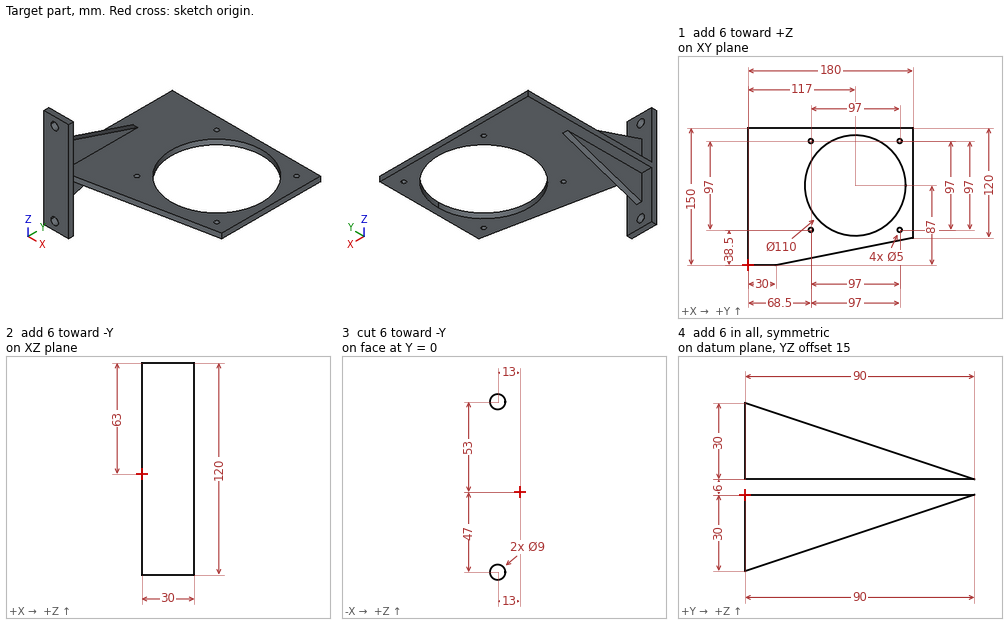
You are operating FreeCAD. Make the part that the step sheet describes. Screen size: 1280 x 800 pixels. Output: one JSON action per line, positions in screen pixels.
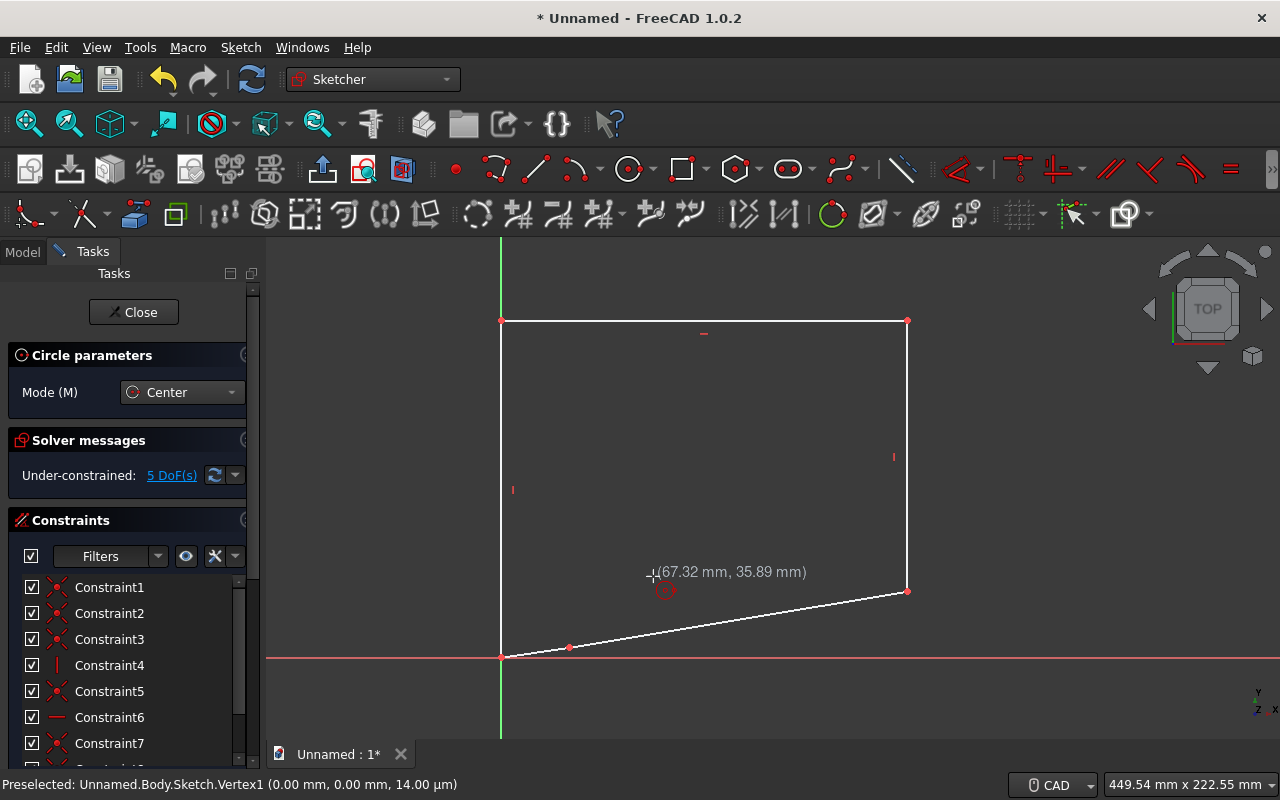
{"action": "left_click", "coordinate": [656, 571]}
{"action": "mouse_move", "coordinate": [660, 567]}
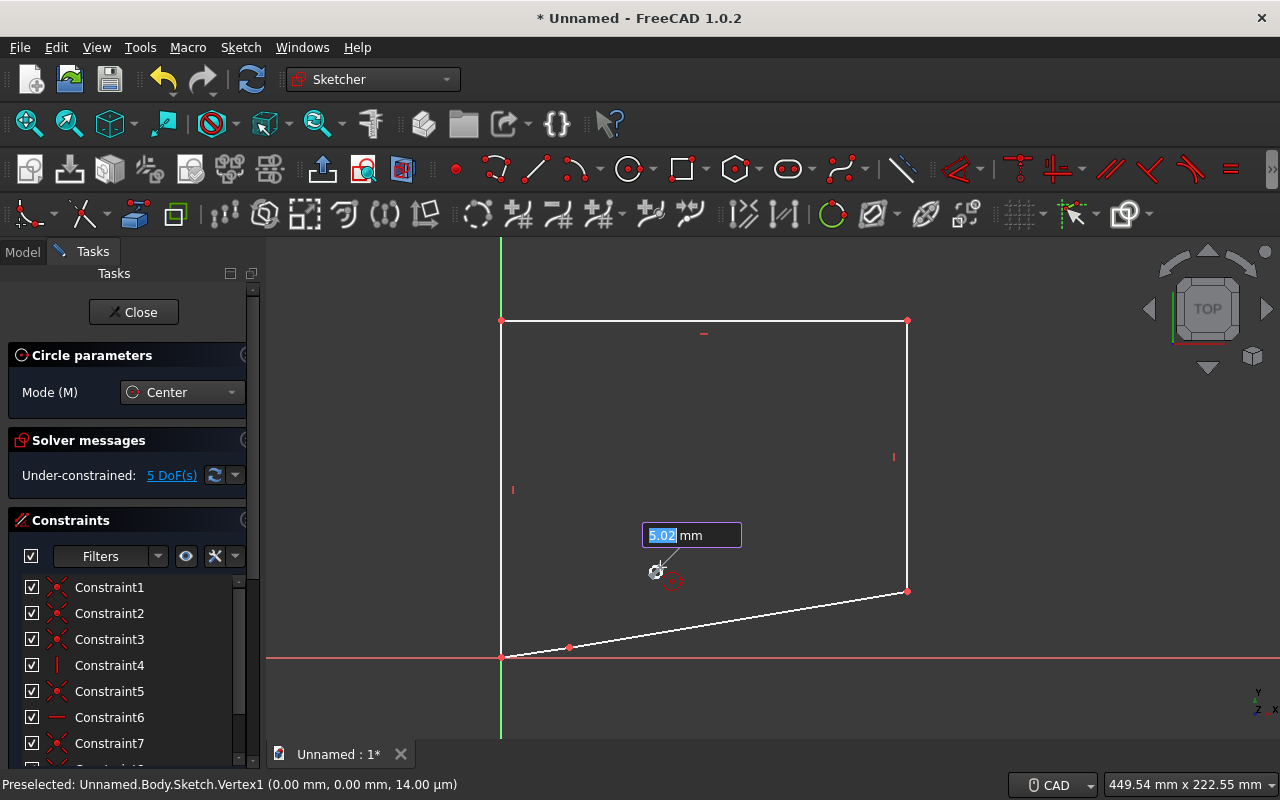
{"action": "type", "text": "5"}
{"action": "key", "text": "Return"}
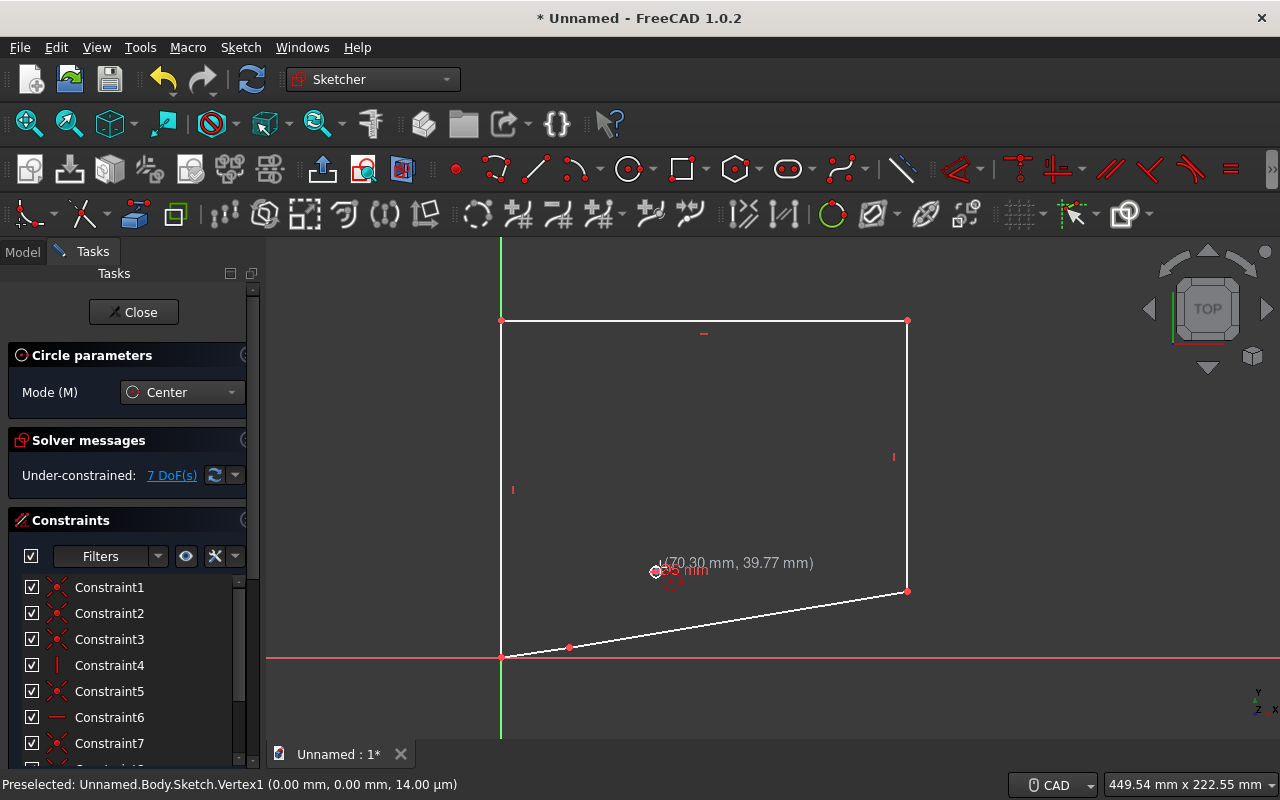
{"action": "scroll", "coordinate": [875, 571], "scroll_direction": "up", "scroll_amount": 7}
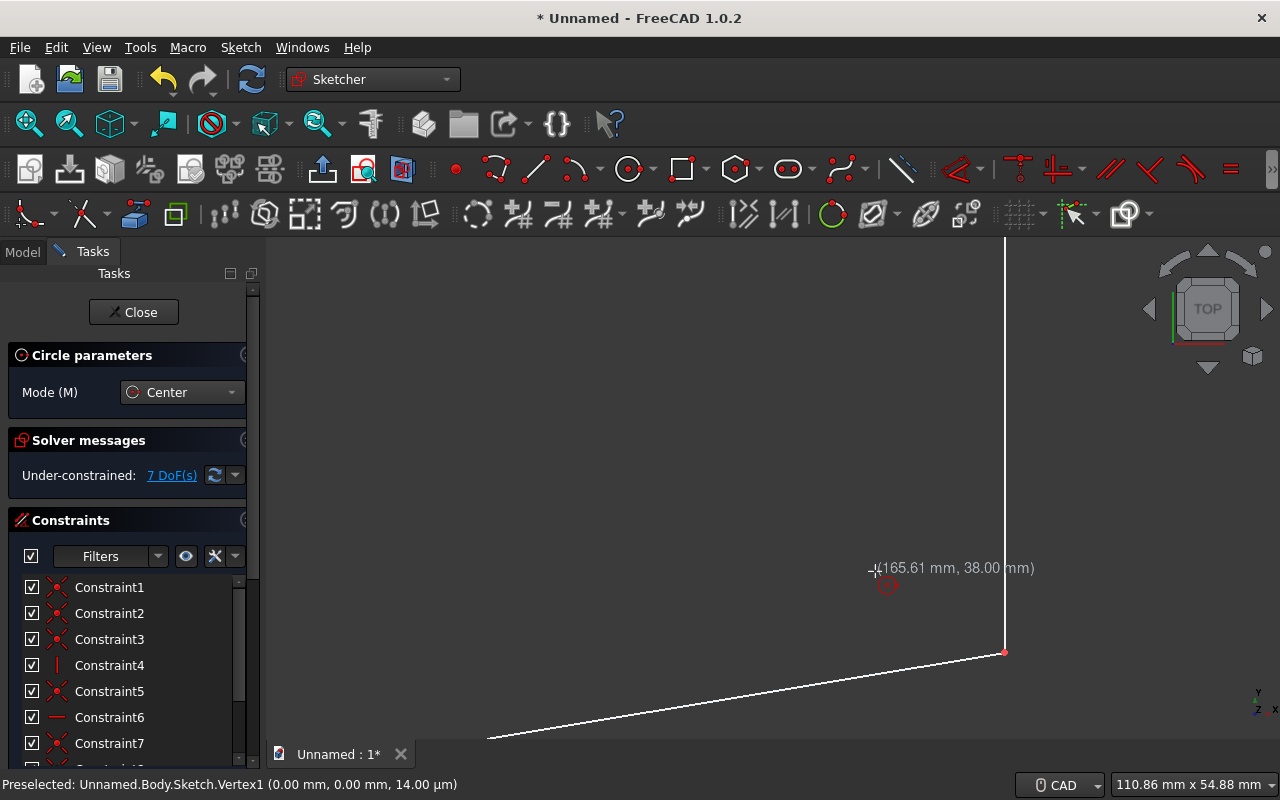
{"action": "scroll", "coordinate": [876, 571], "scroll_direction": "down", "scroll_amount": 7}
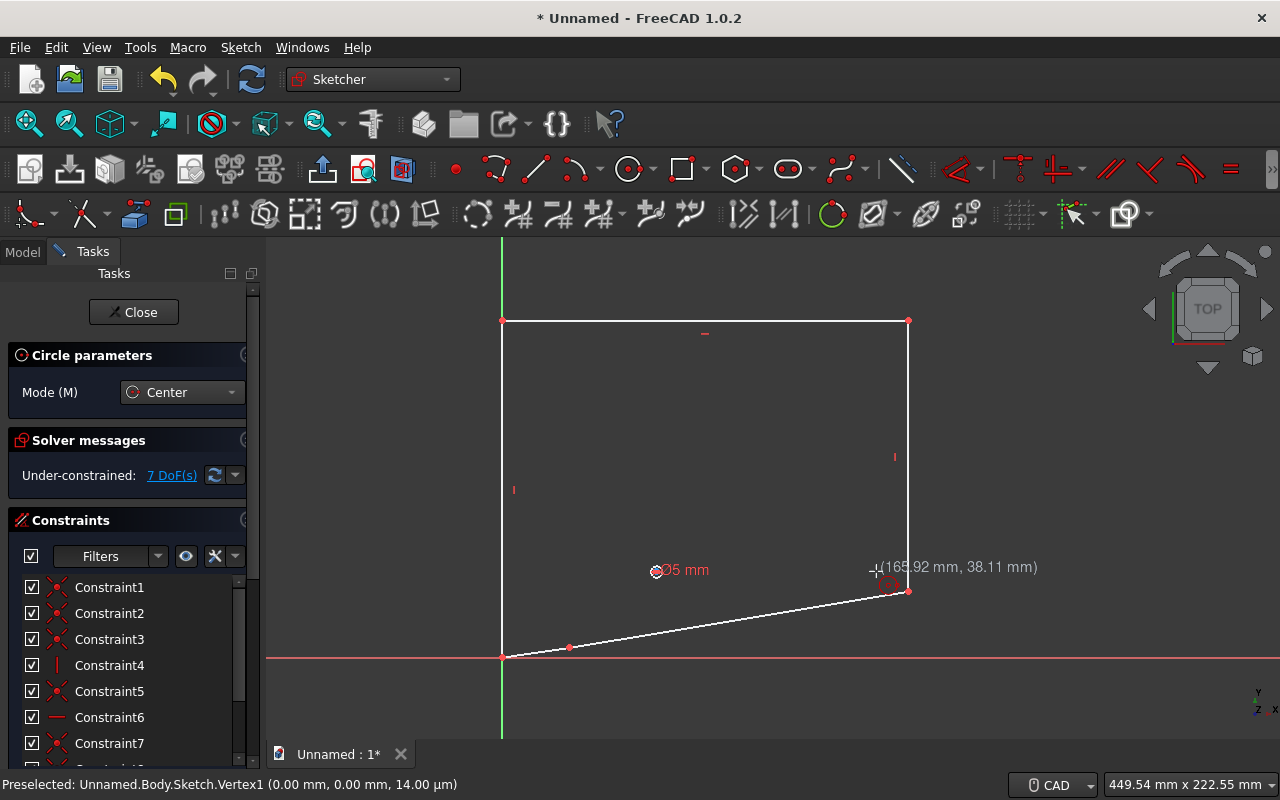
{"action": "left_click", "coordinate": [875, 571]}
{"action": "mouse_move", "coordinate": [879, 567]}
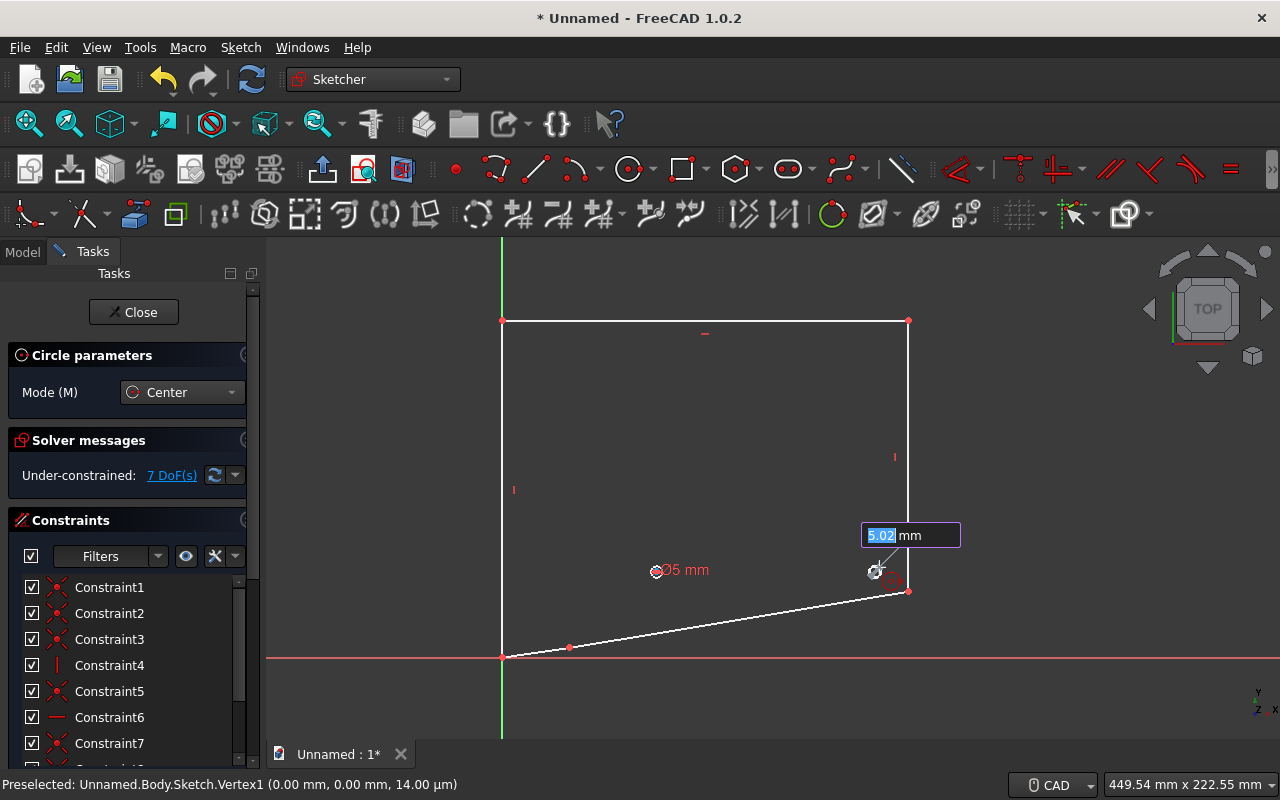
{"action": "type", "text": "5"}
{"action": "key", "text": "Return"}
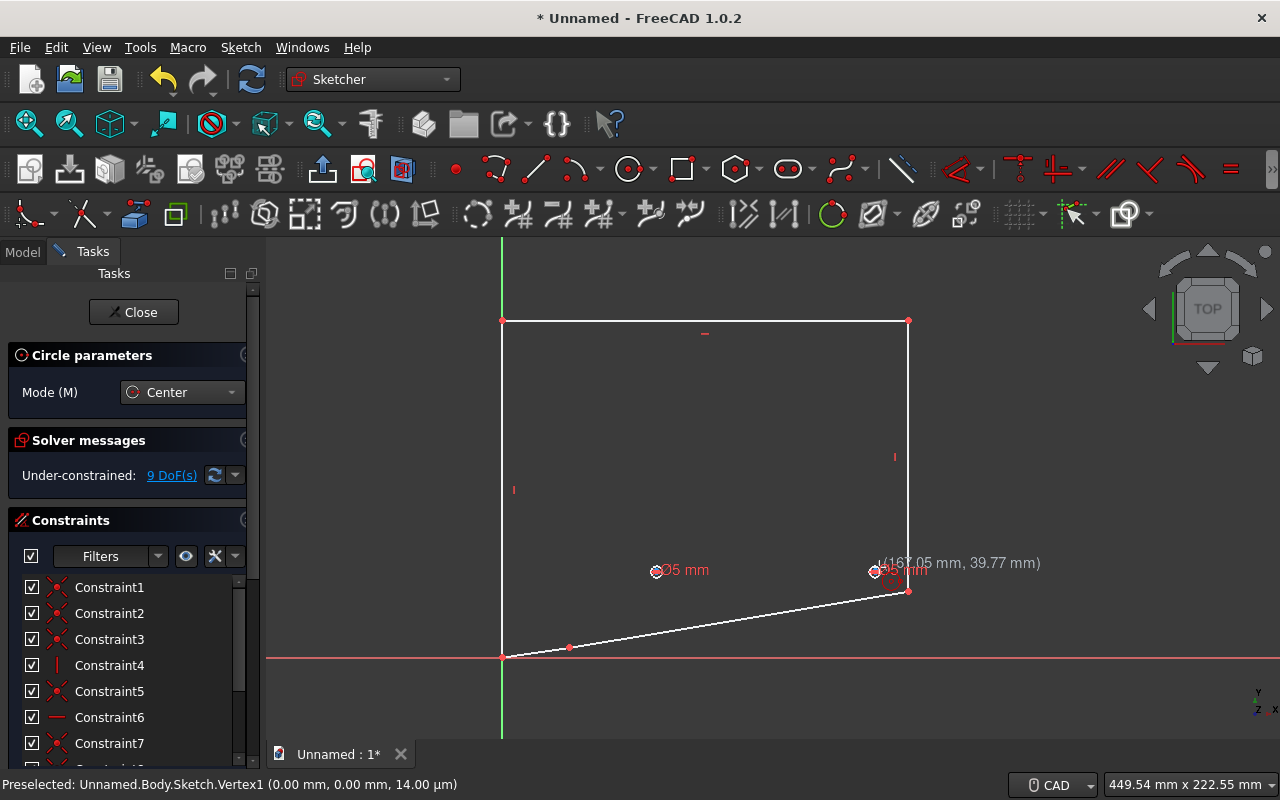
{"action": "scroll", "coordinate": [657, 352], "scroll_direction": "up", "scroll_amount": 7}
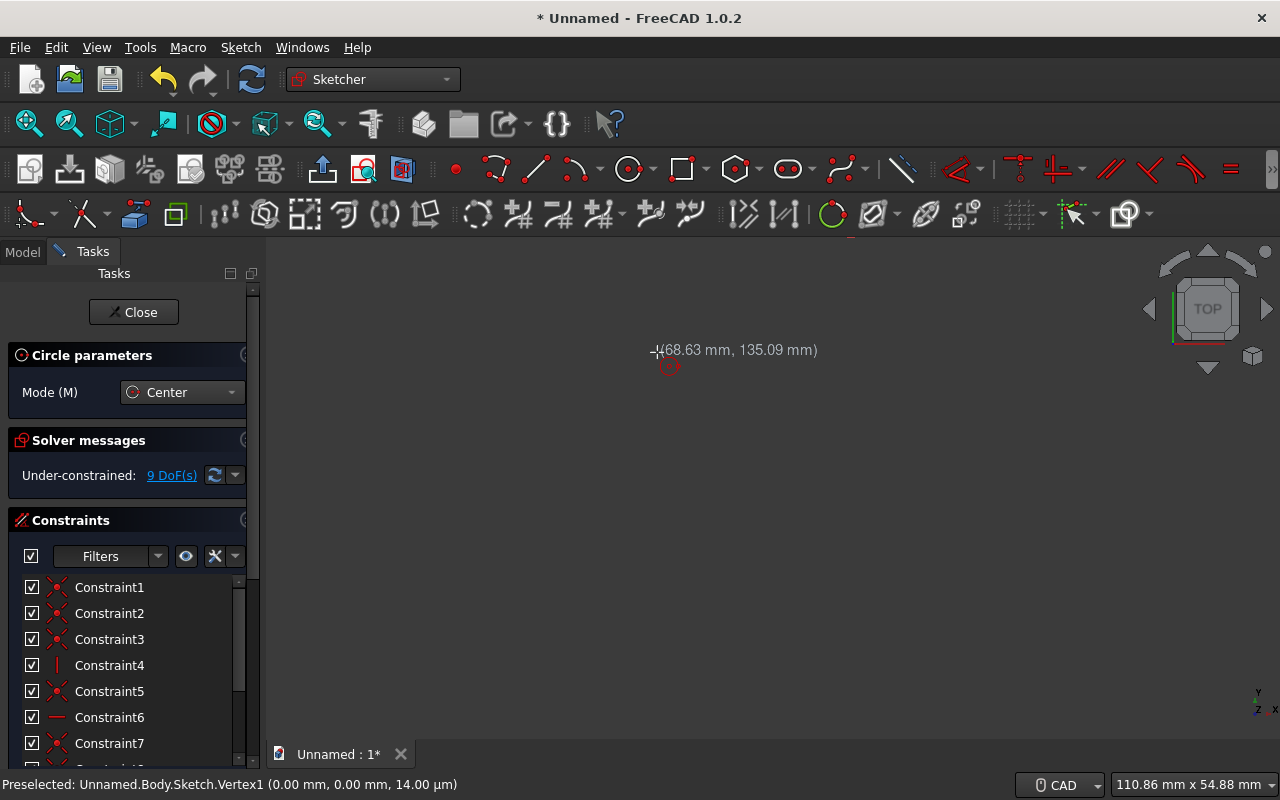
{"action": "scroll", "coordinate": [656, 352], "scroll_direction": "down", "scroll_amount": 7}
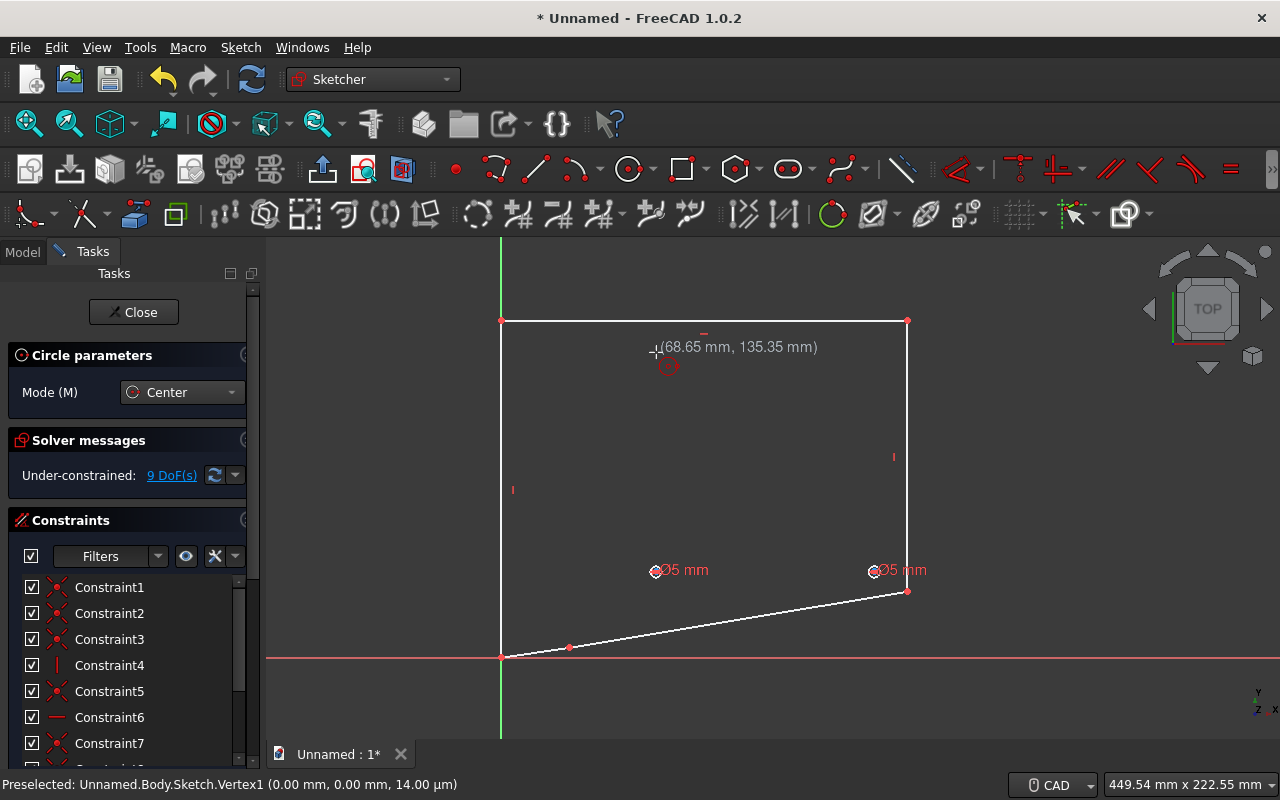
{"action": "left_click", "coordinate": [656, 352]}
{"action": "mouse_move", "coordinate": [660, 348]}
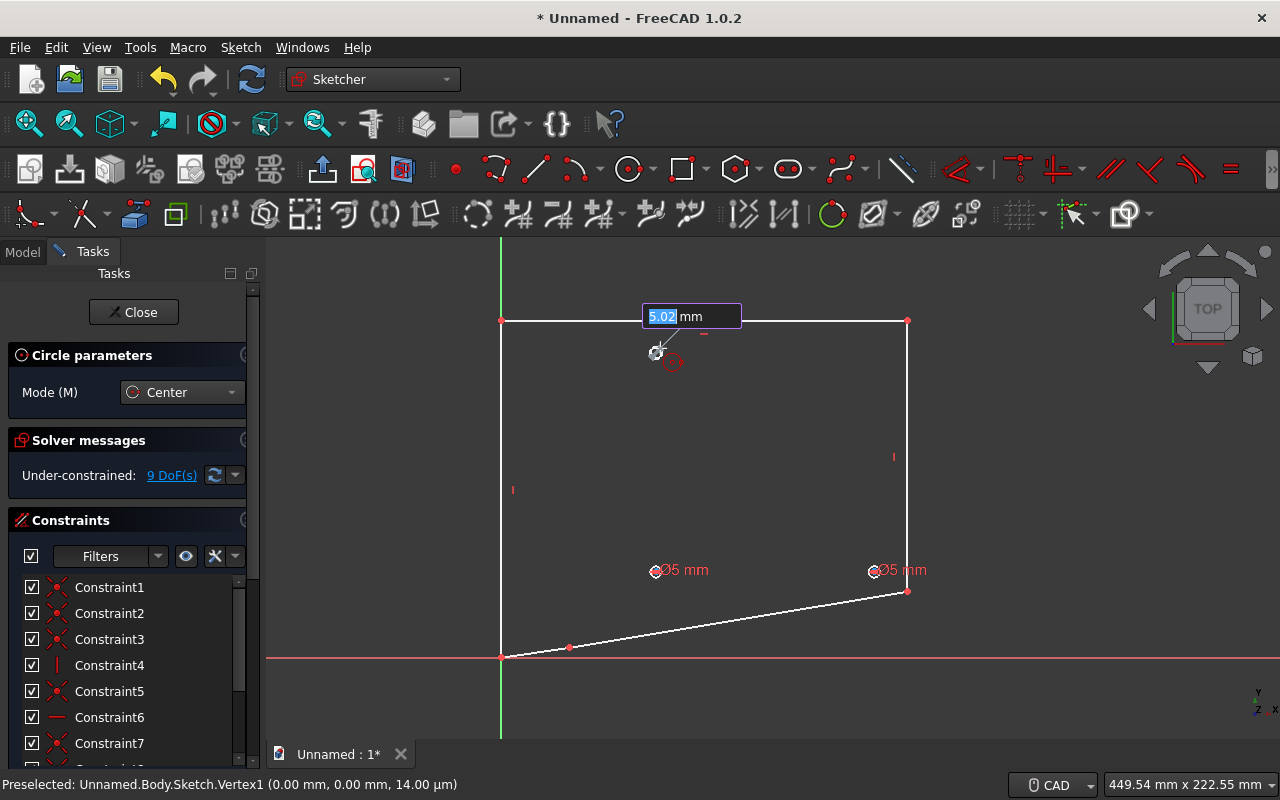
{"action": "type", "text": "5"}
{"action": "key", "text": "Return"}